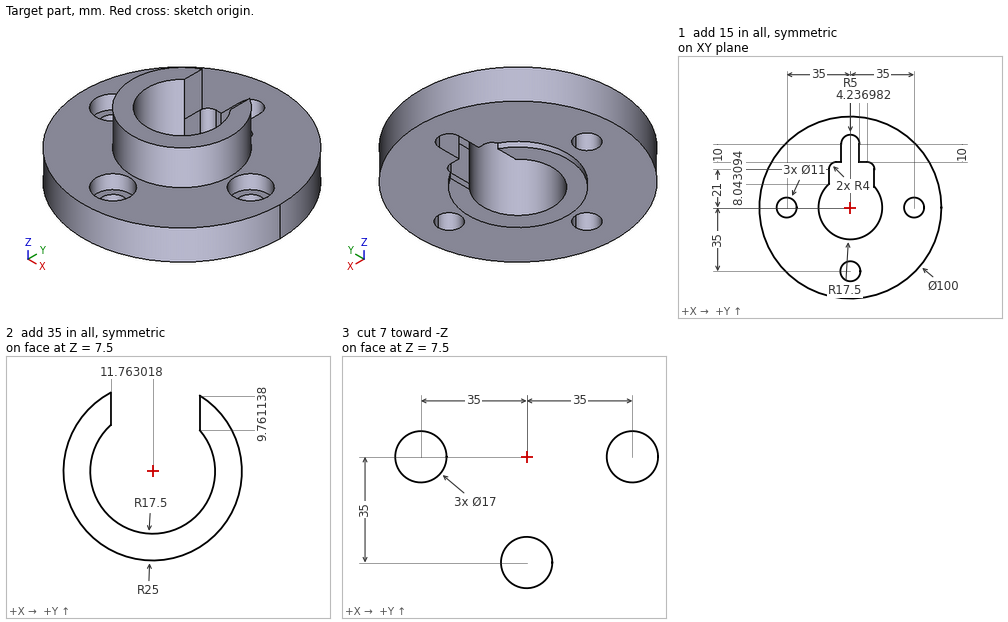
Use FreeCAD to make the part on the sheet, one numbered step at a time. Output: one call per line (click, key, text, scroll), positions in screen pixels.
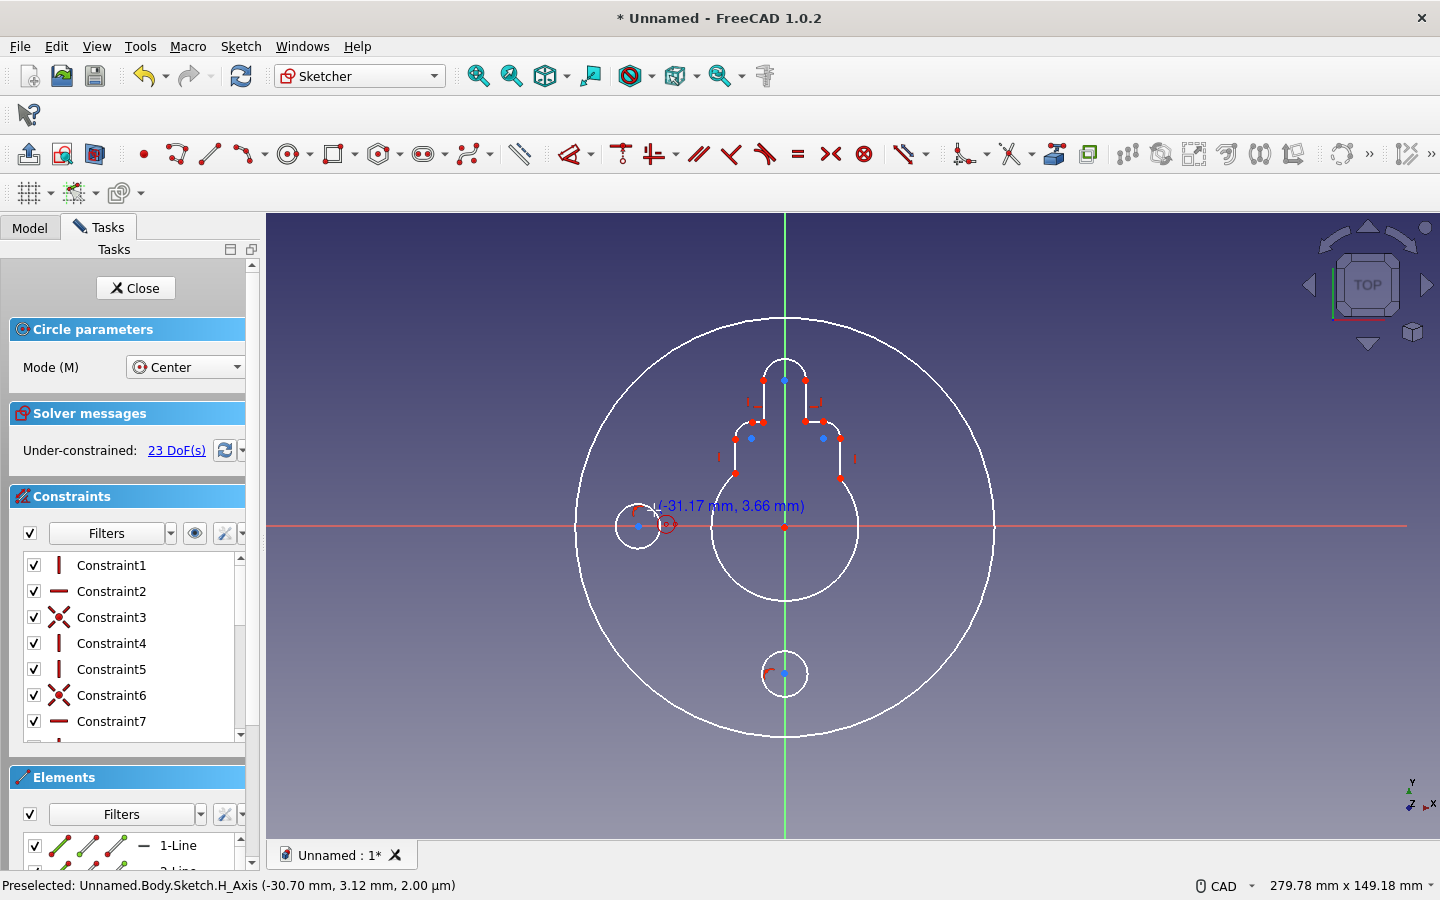
click(932, 526)
click(948, 510)
key(Escape)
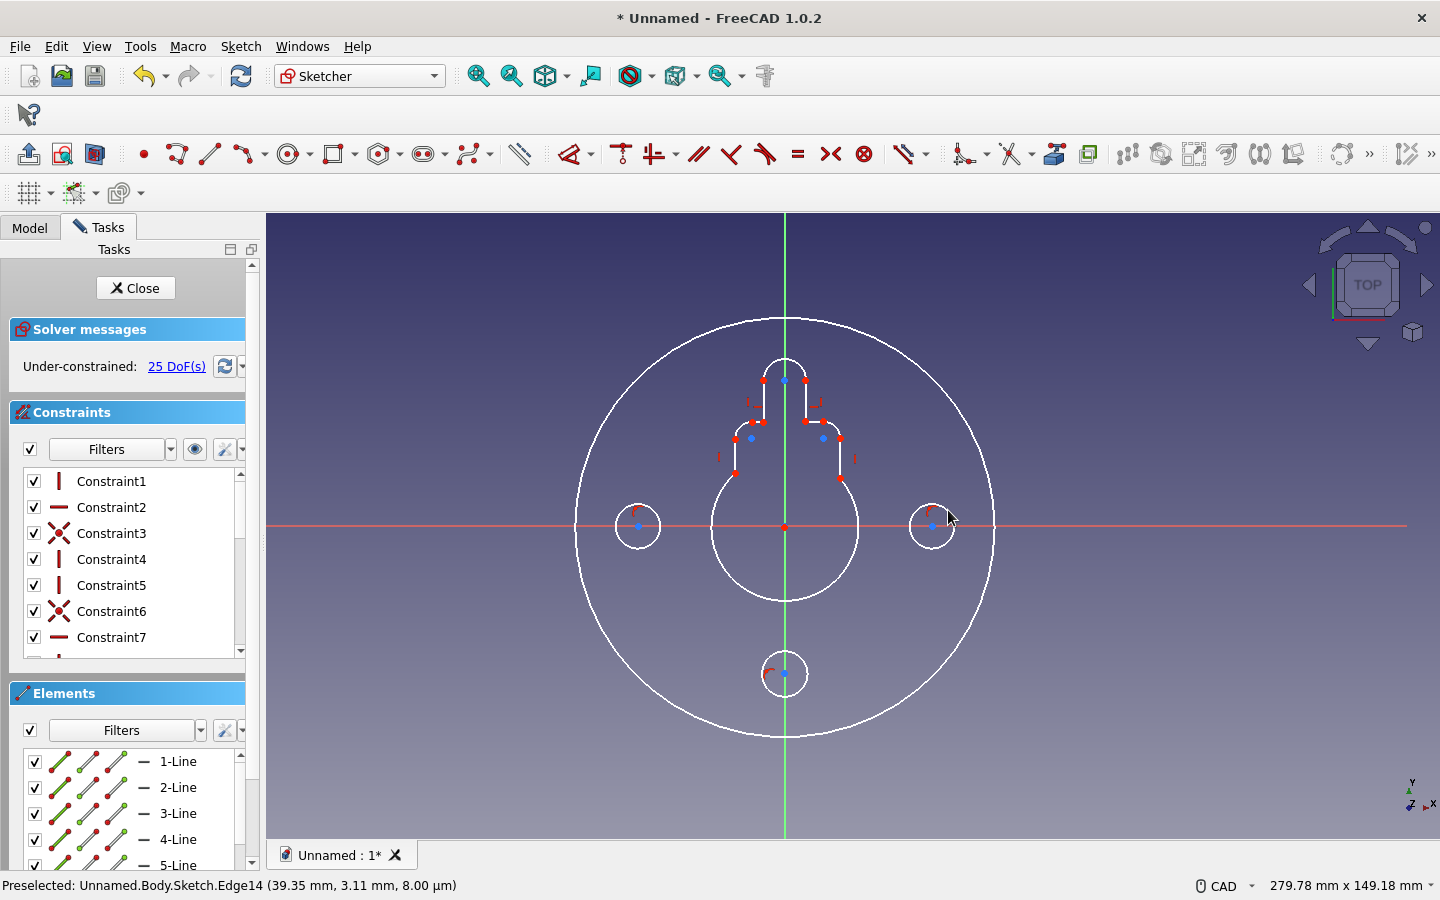
scroll(735, 463, up, 2)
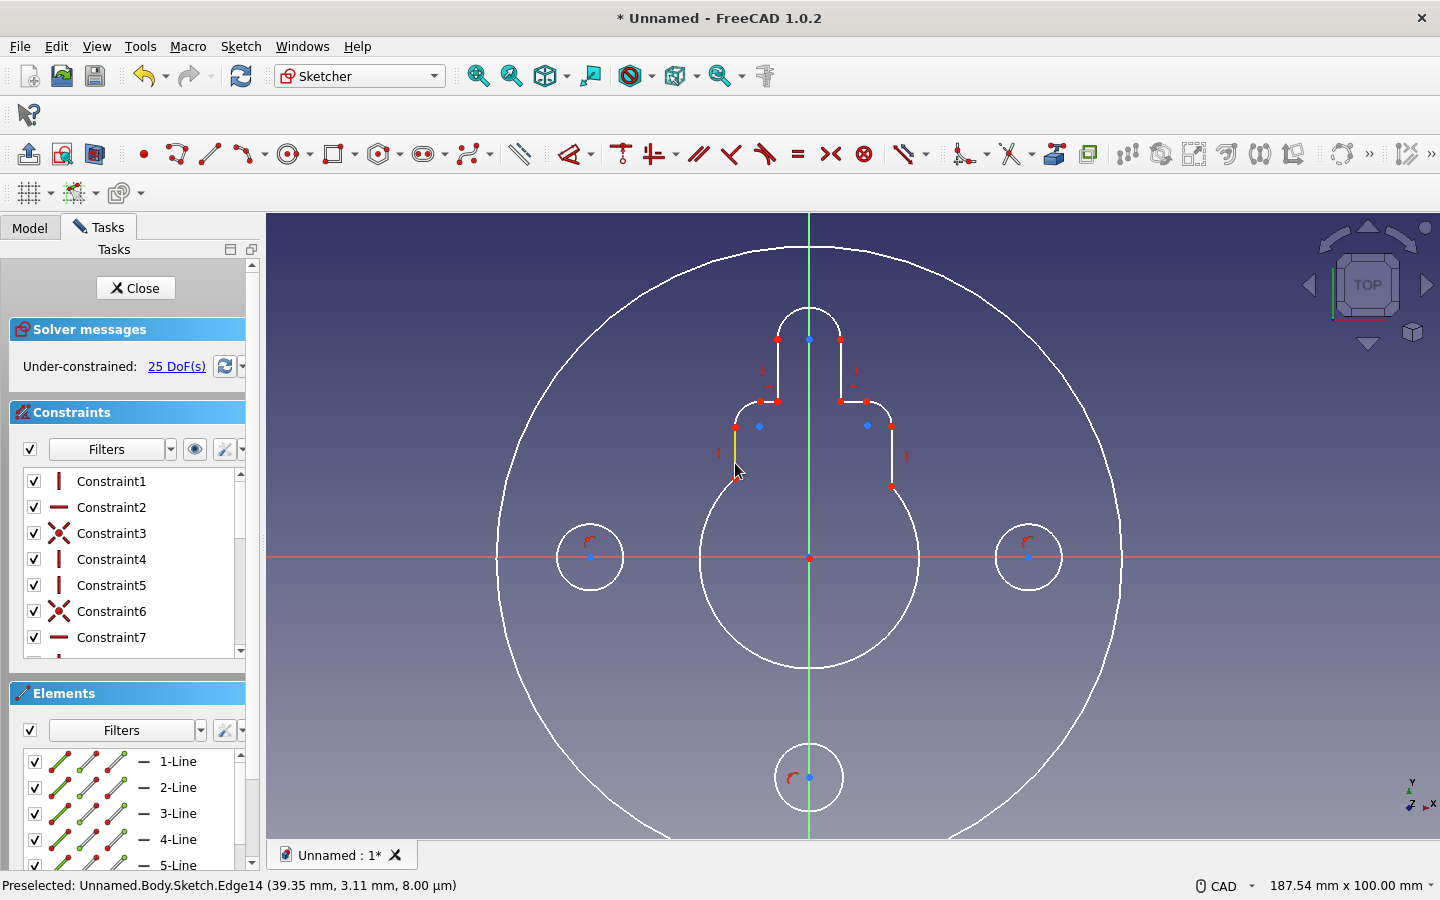
click(735, 463)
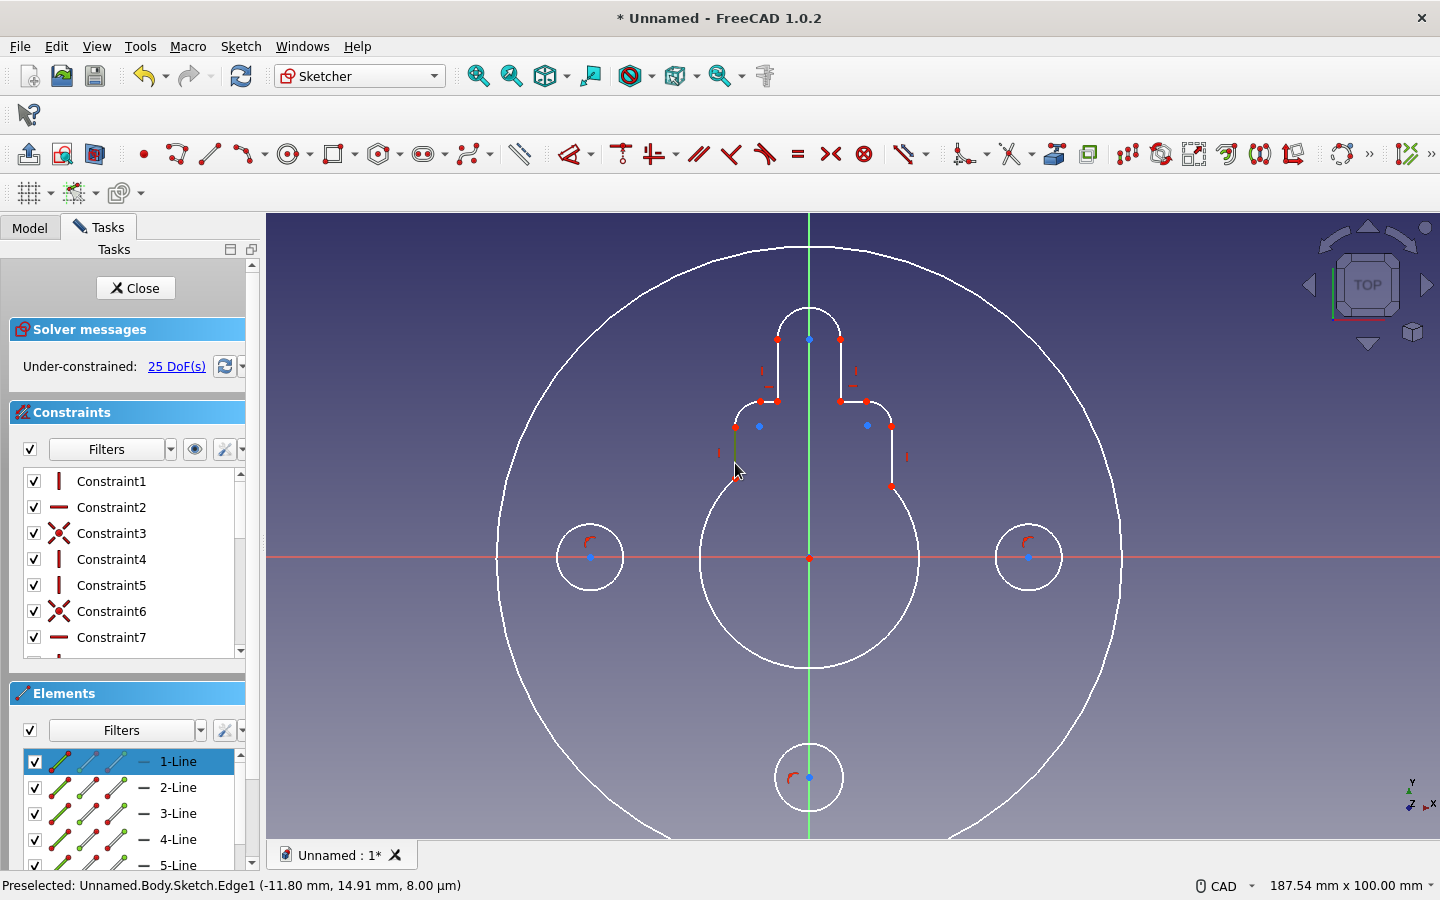
click(749, 404)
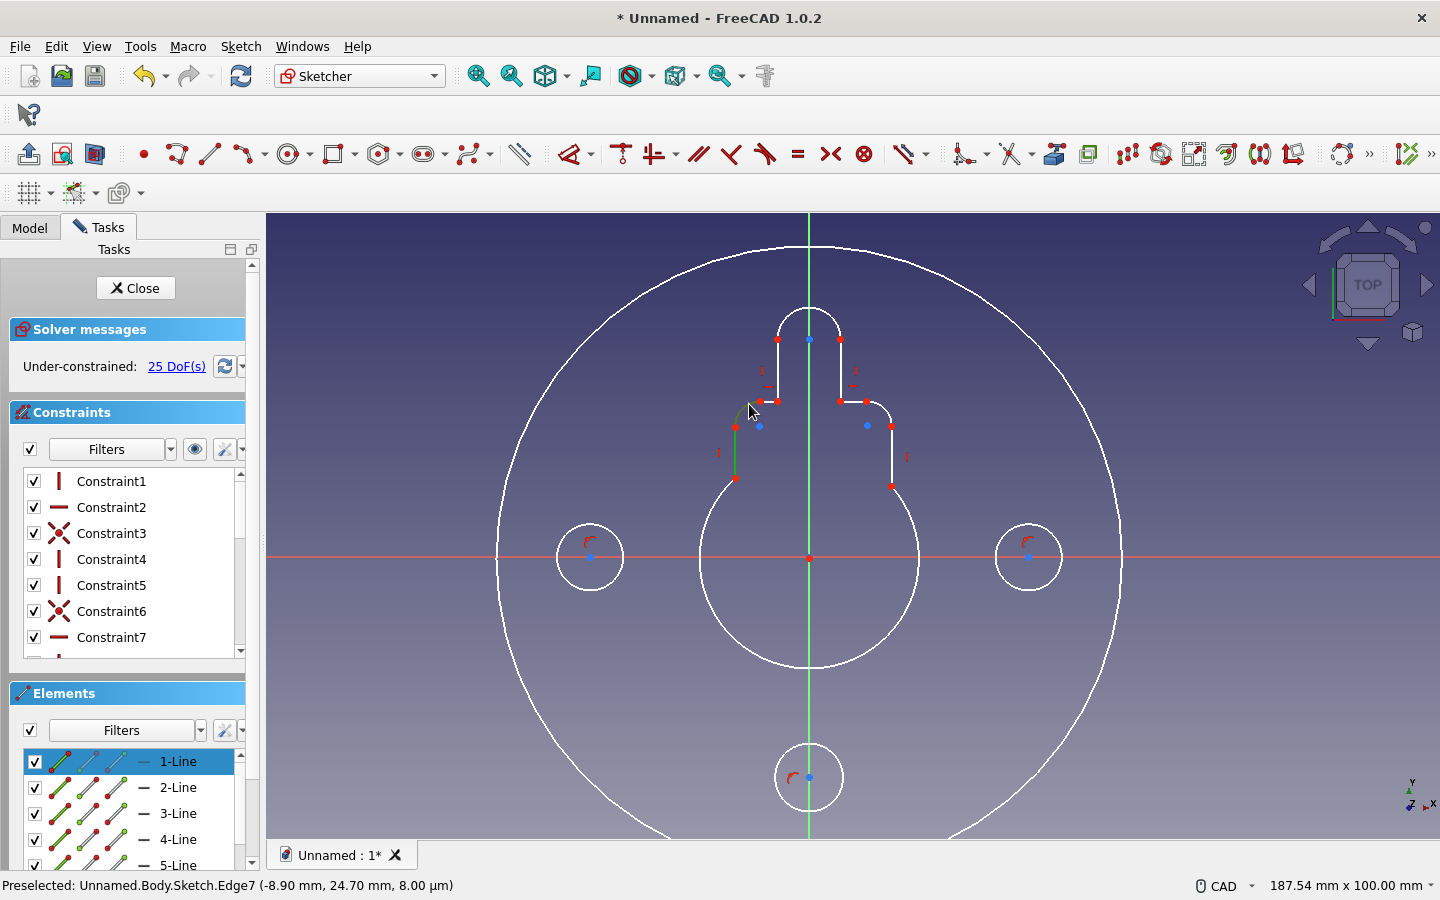
key(t)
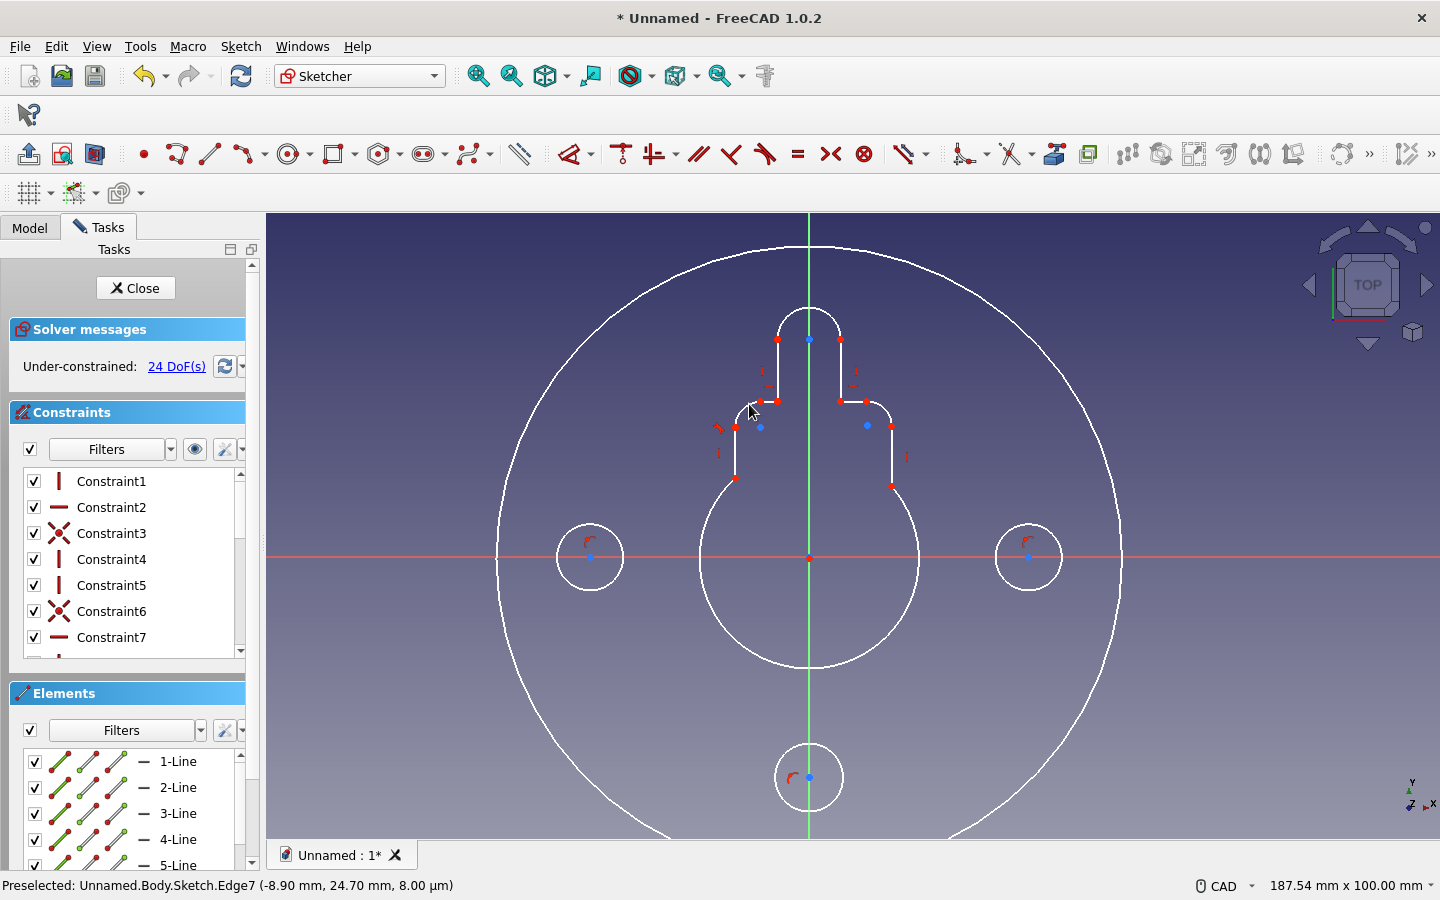
scroll(769, 402, up, 3)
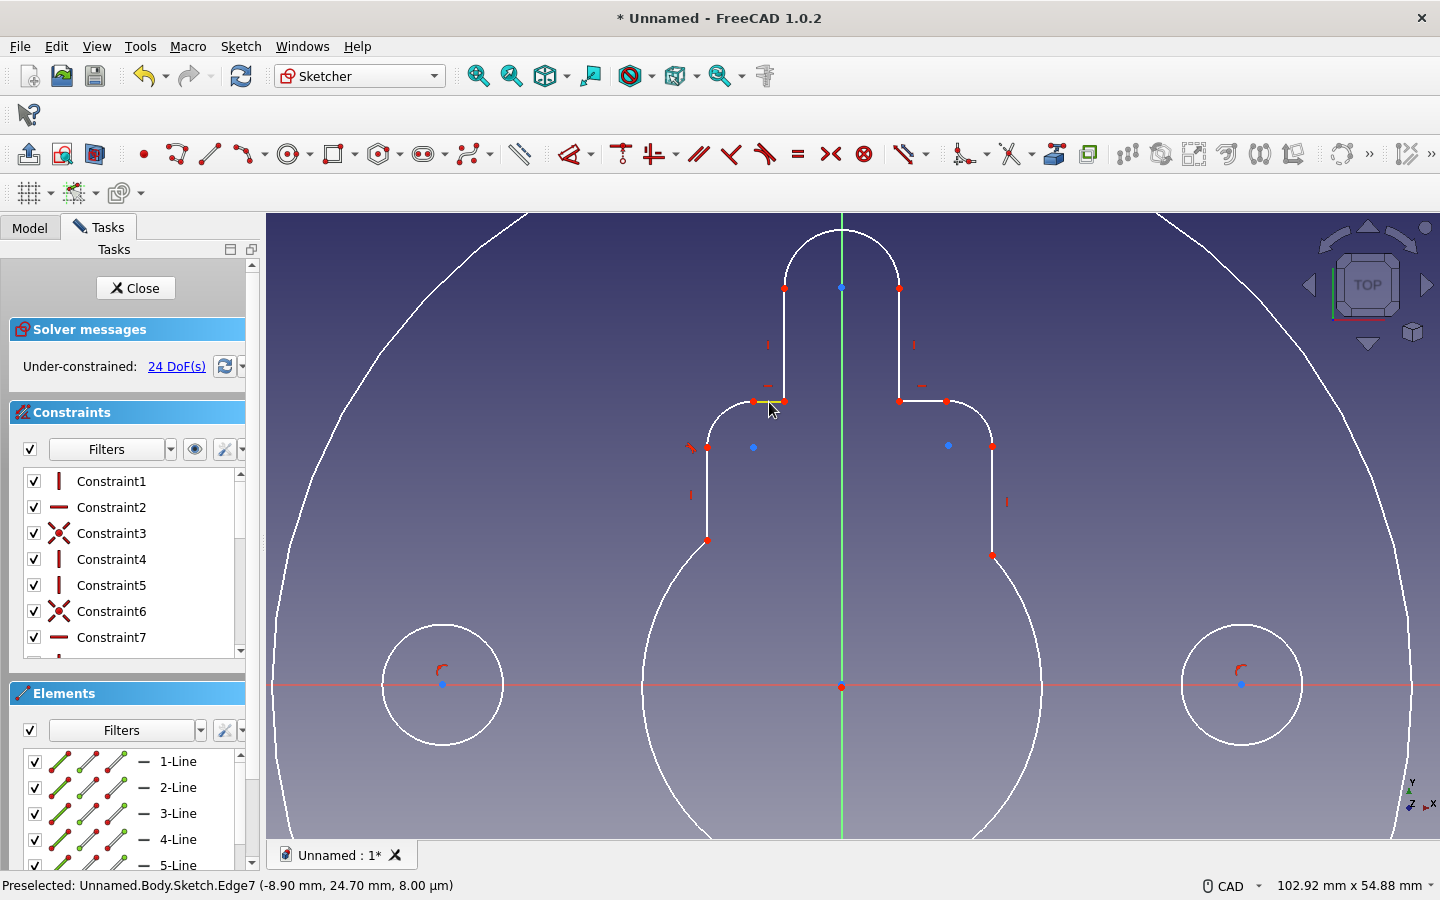
click(769, 402)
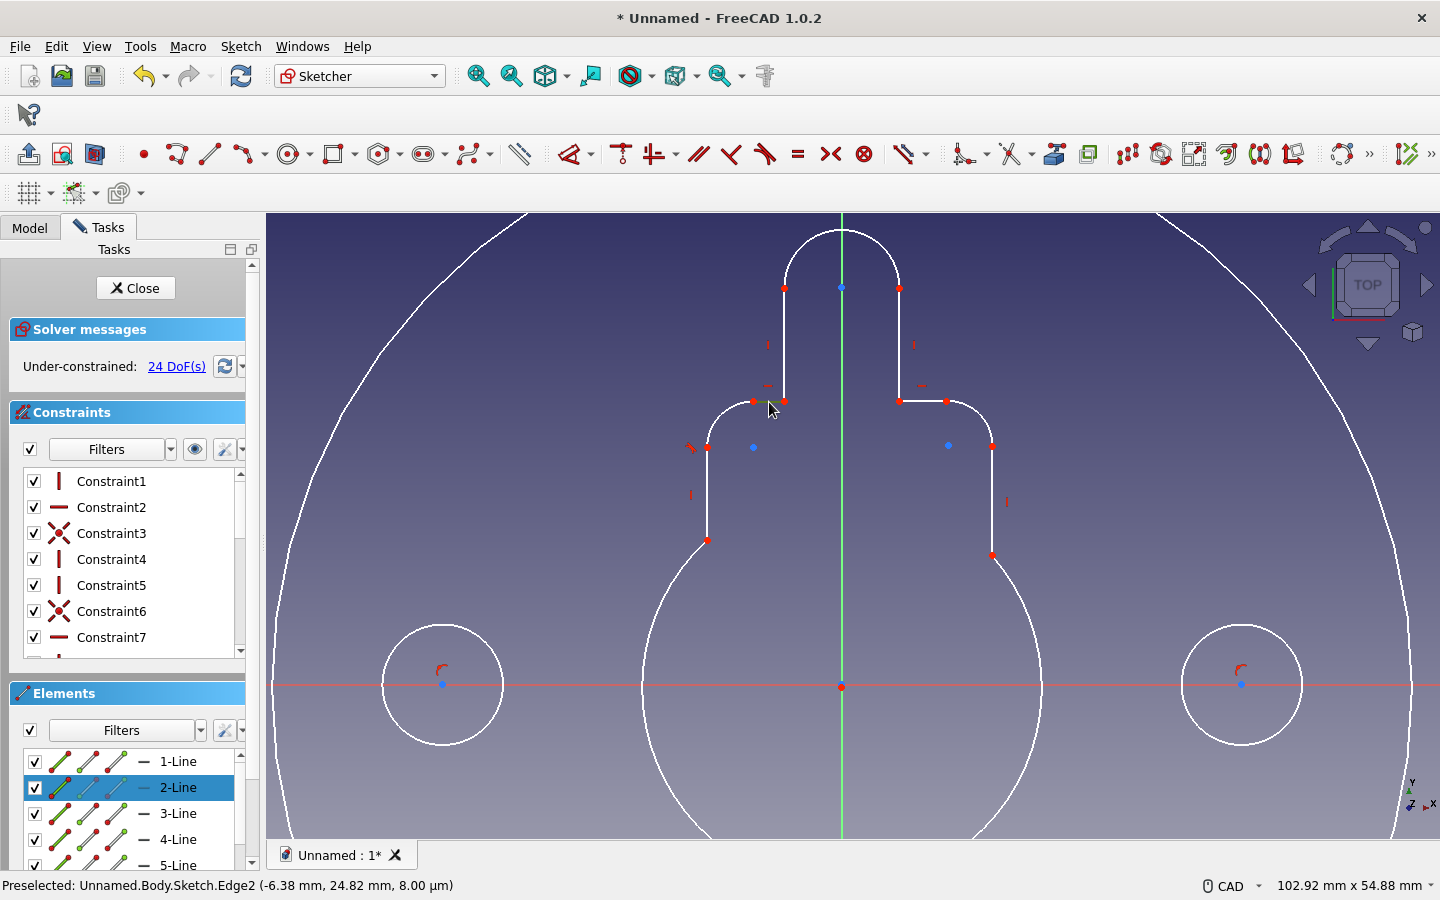
click(732, 407)